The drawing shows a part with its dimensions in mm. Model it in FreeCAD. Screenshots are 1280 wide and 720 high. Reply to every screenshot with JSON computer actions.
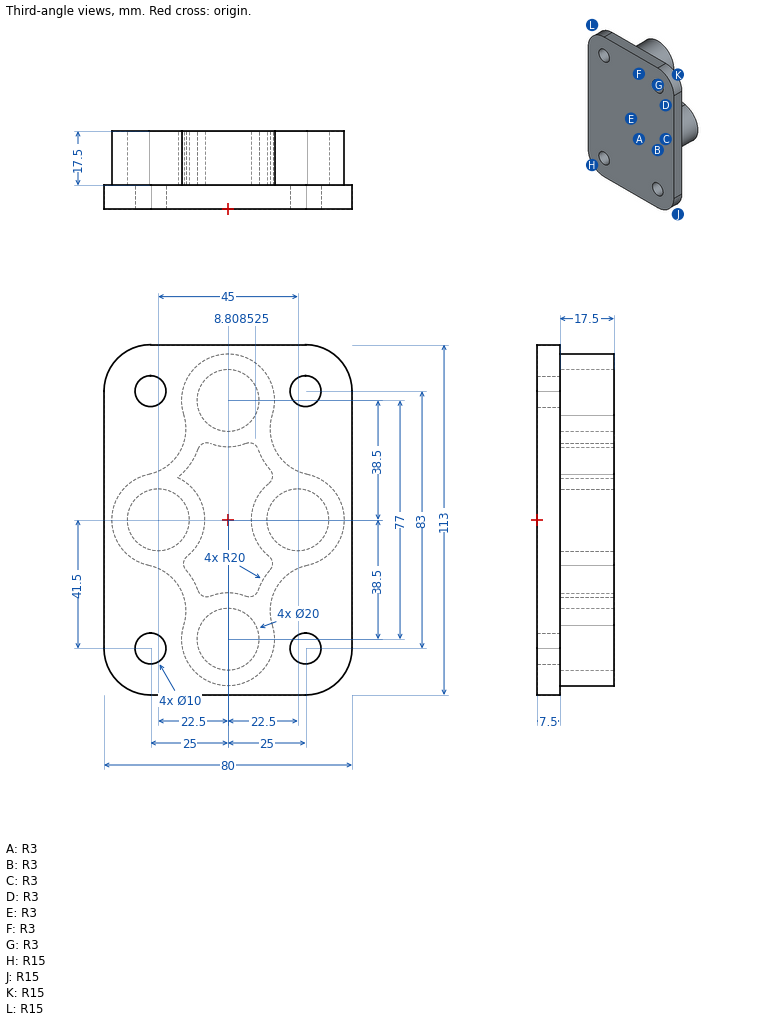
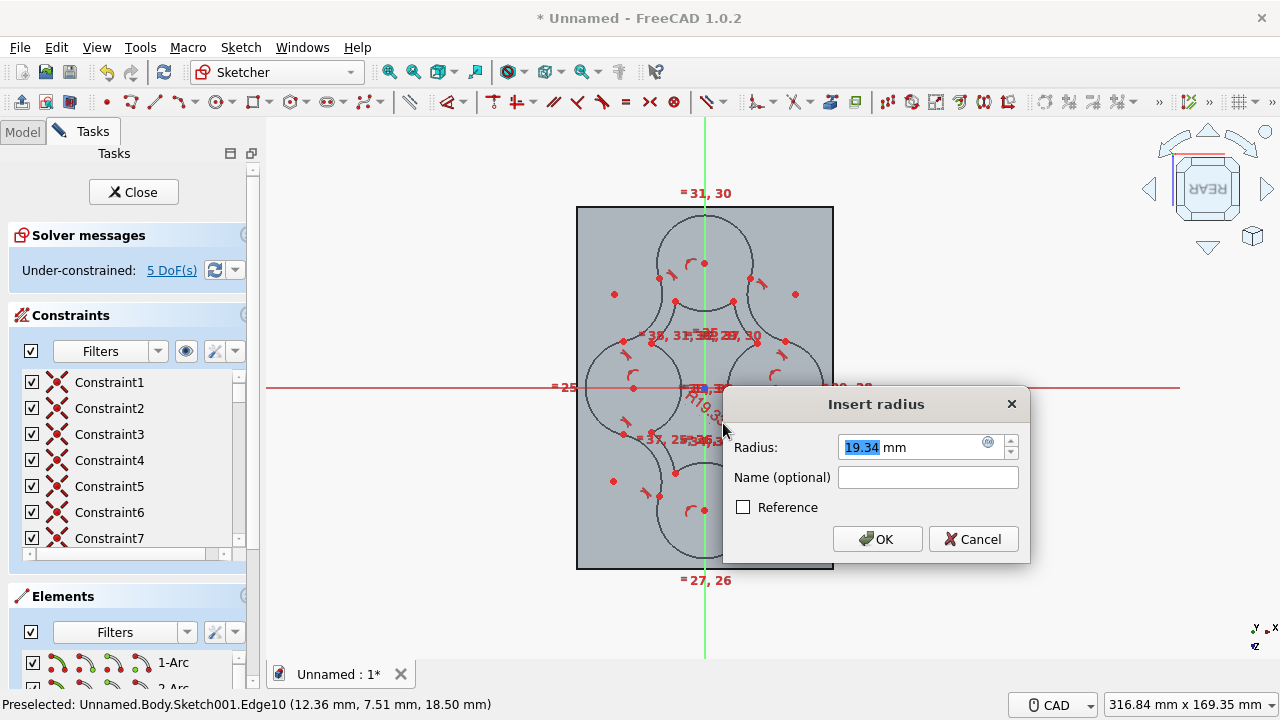
{"action": "type", "text": "20"}
{"action": "key", "text": "Return"}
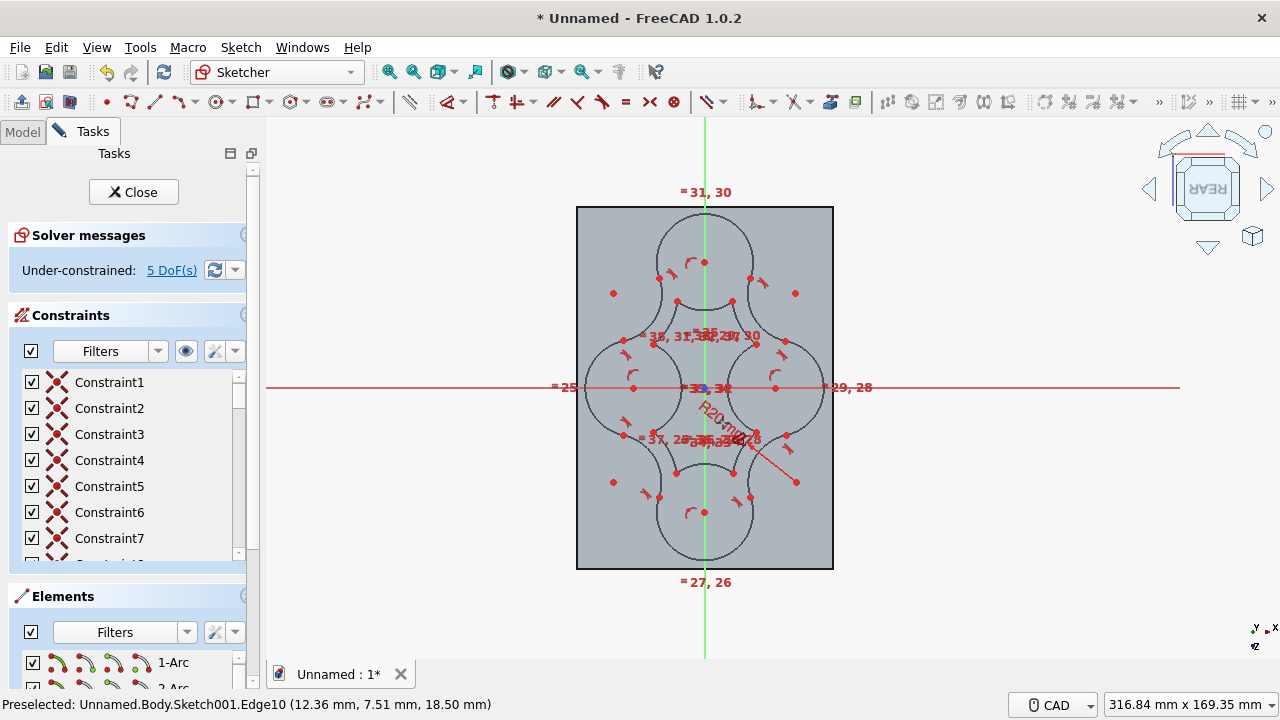
{"action": "left_click", "coordinate": [633, 388]}
{"action": "left_click", "coordinate": [644, 422]}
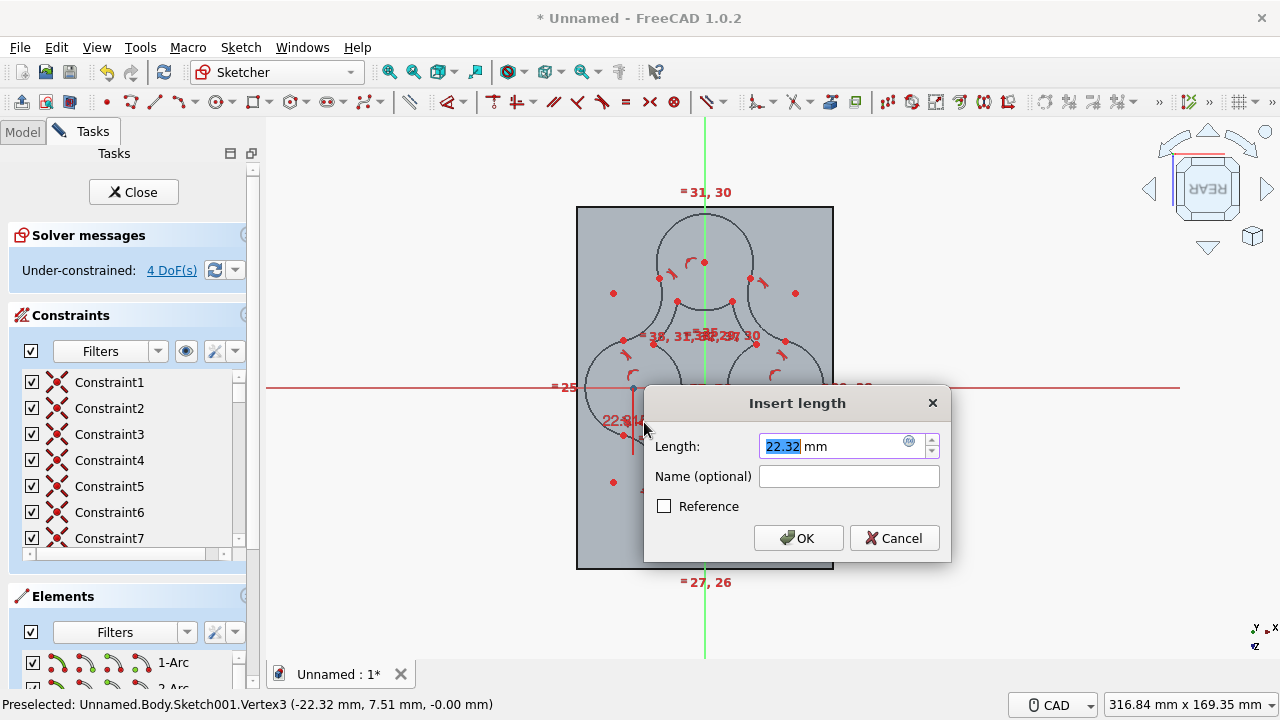
{"action": "type", "text": "22.5"}
{"action": "key", "text": "Return"}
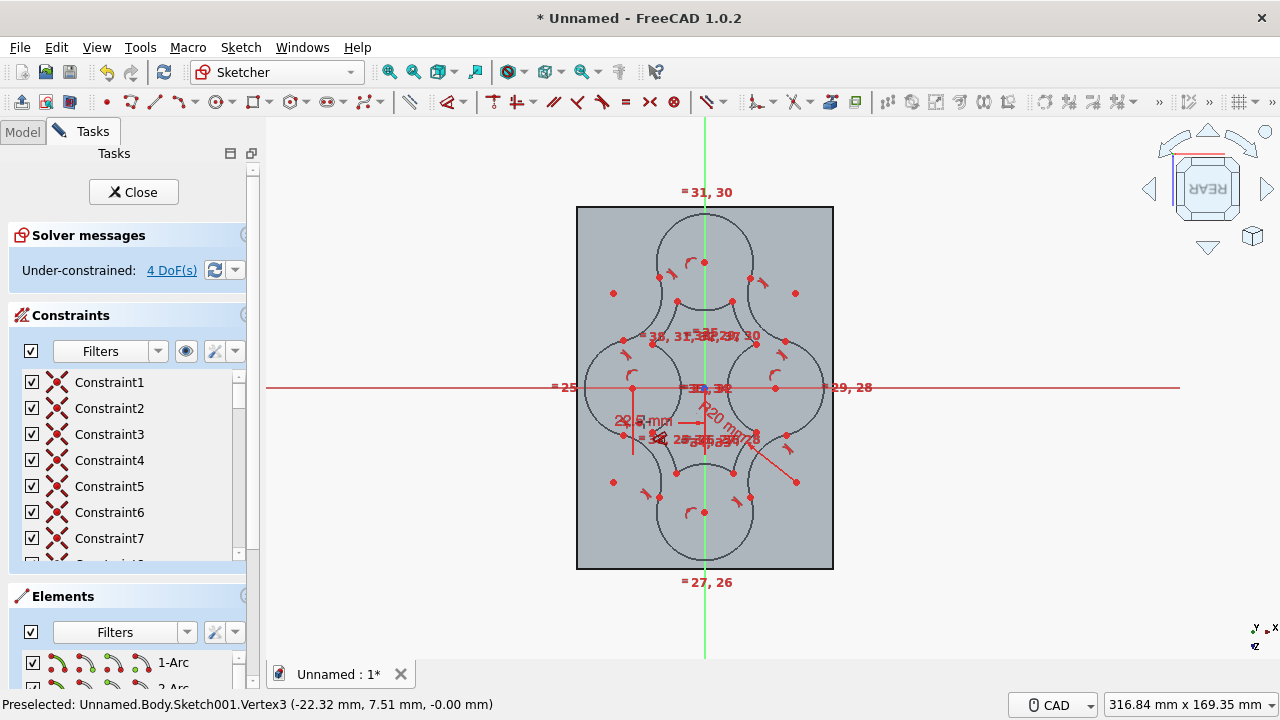
{"action": "left_click", "coordinate": [705, 512]}
{"action": "left_click", "coordinate": [763, 479]}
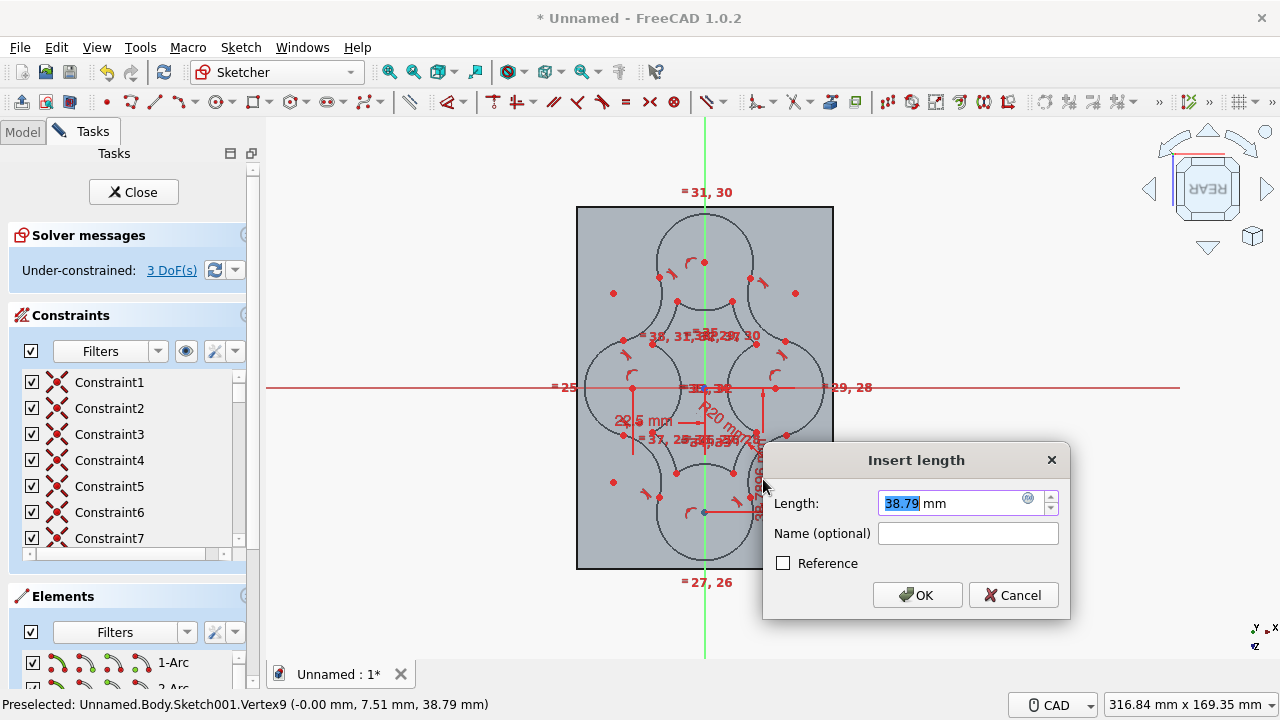
{"action": "type", "text": "38.5"}
{"action": "key", "text": "Return"}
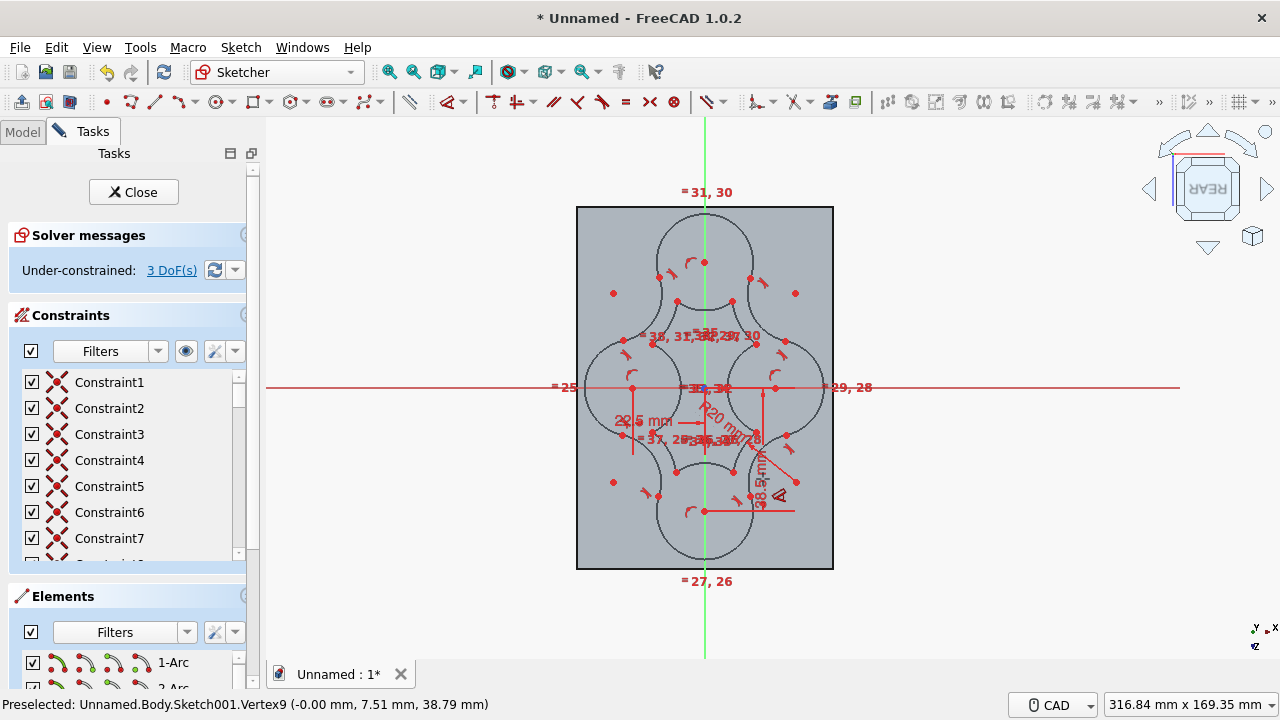
{"action": "left_click", "coordinate": [776, 388]}
{"action": "left_click", "coordinate": [724, 354]}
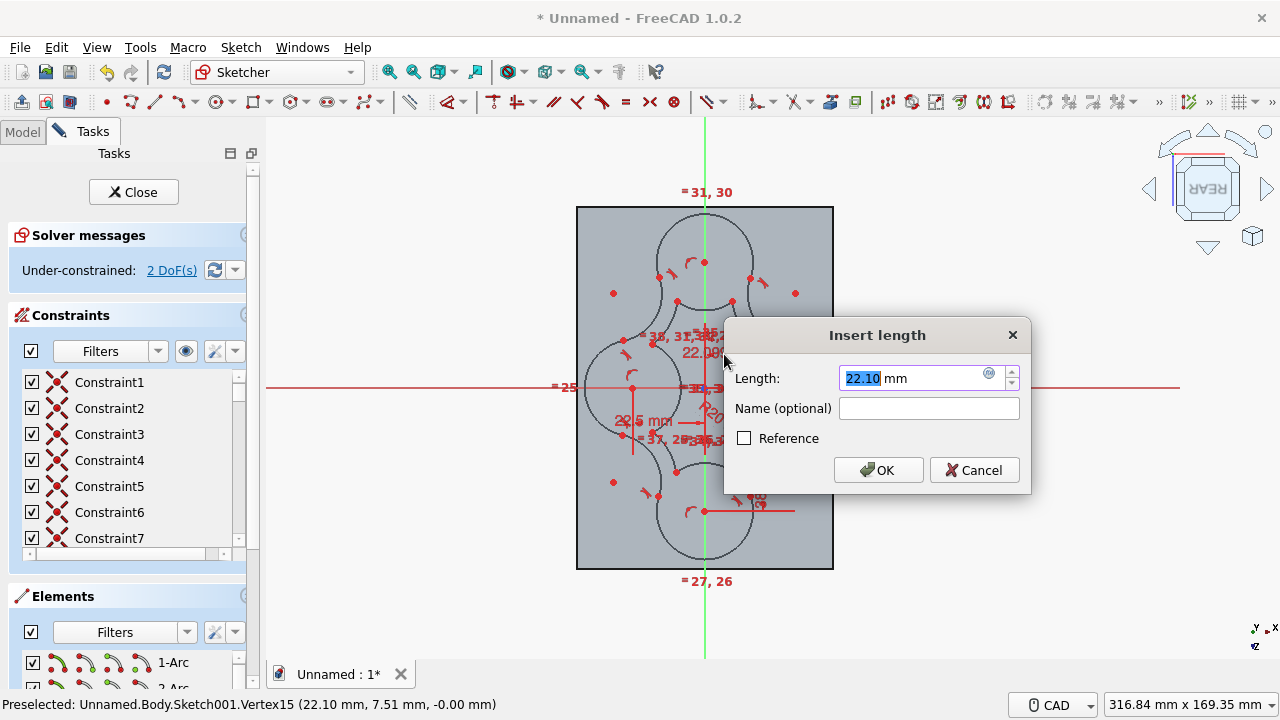
{"action": "type", "text": "22.5"}
{"action": "key", "text": "Return"}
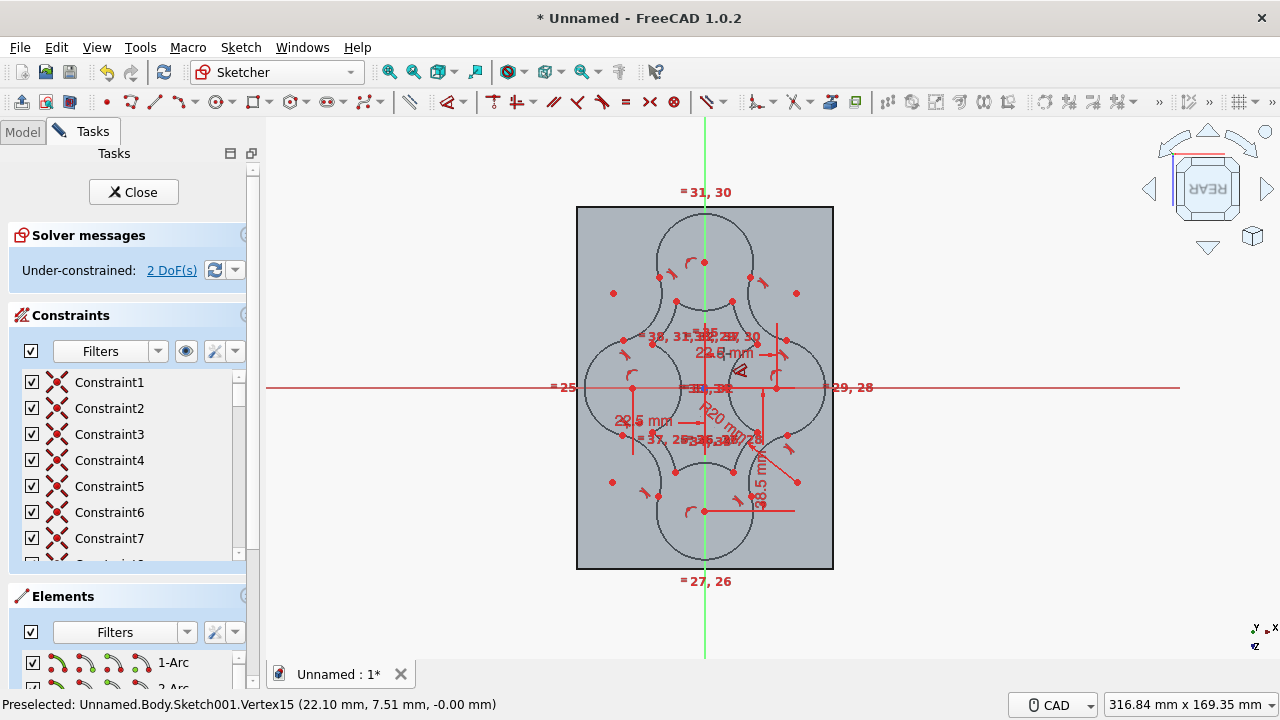
{"action": "left_click", "coordinate": [705, 262]}
{"action": "left_click", "coordinate": [763, 296]}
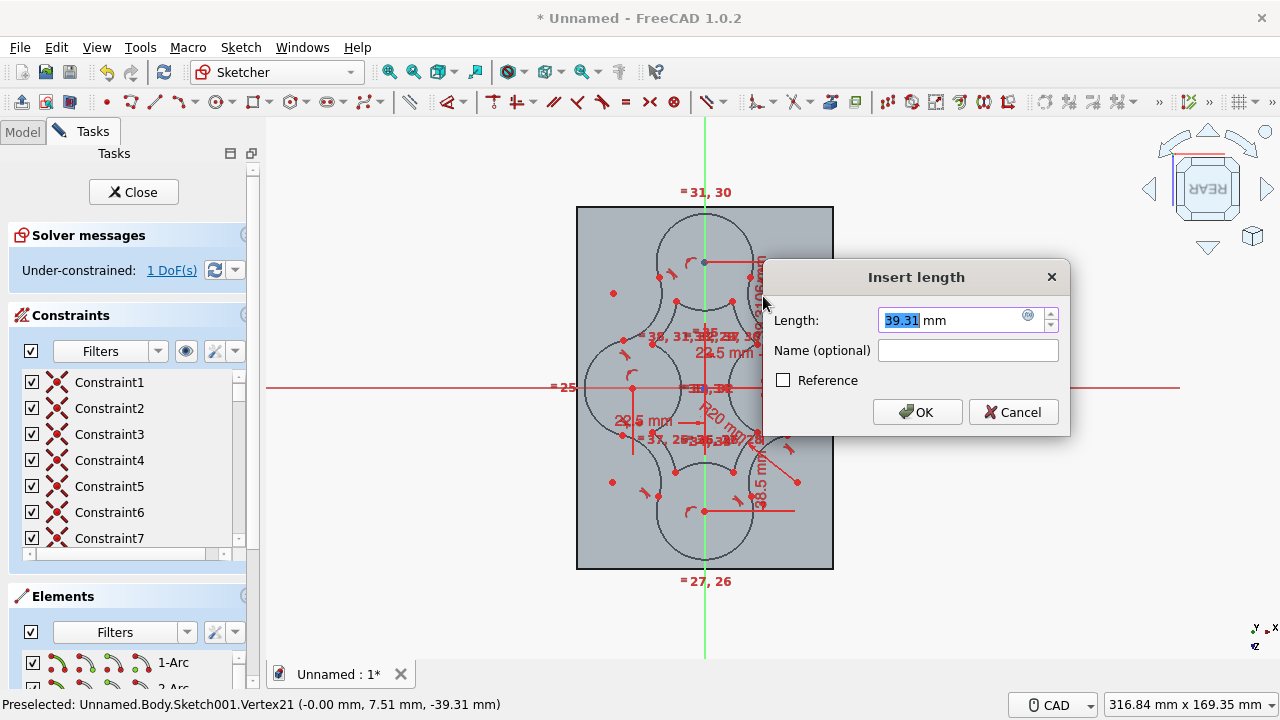
{"action": "type", "text": "38.5"}
{"action": "key", "text": "Return"}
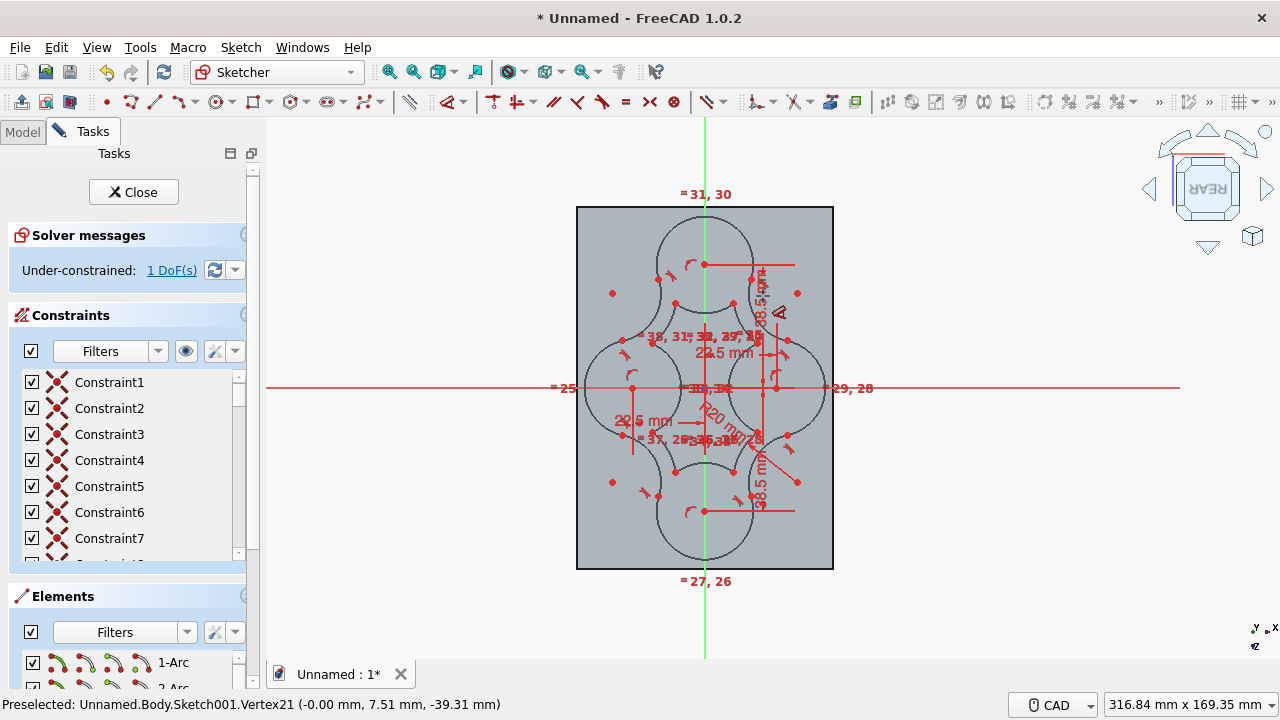
{"action": "scroll", "coordinate": [734, 473], "scroll_direction": "up", "scroll_amount": 2}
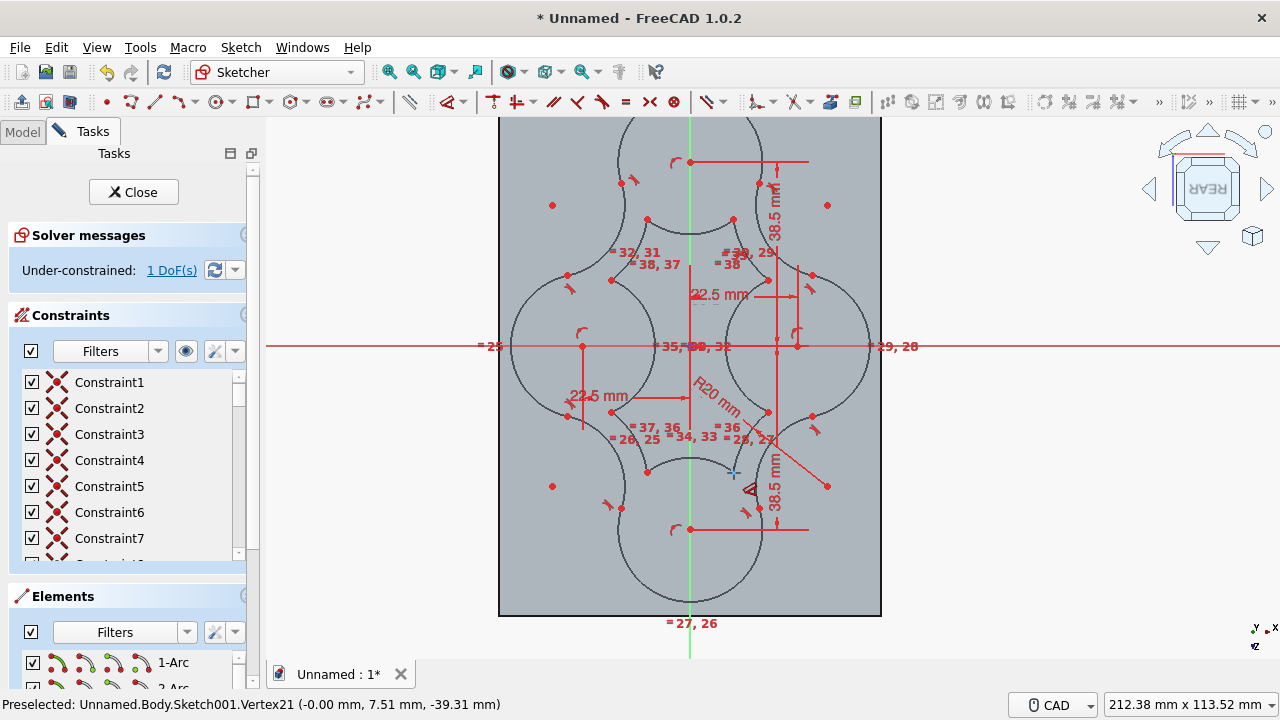
{"action": "left_click", "coordinate": [734, 472]}
{"action": "left_click", "coordinate": [712, 506]}